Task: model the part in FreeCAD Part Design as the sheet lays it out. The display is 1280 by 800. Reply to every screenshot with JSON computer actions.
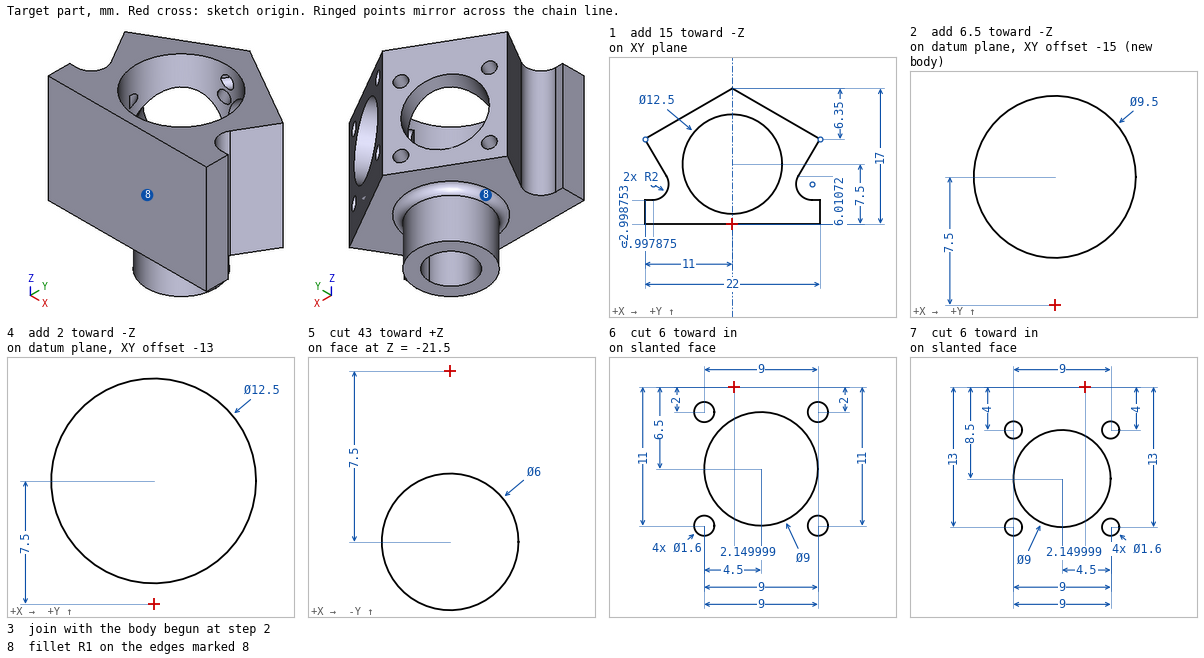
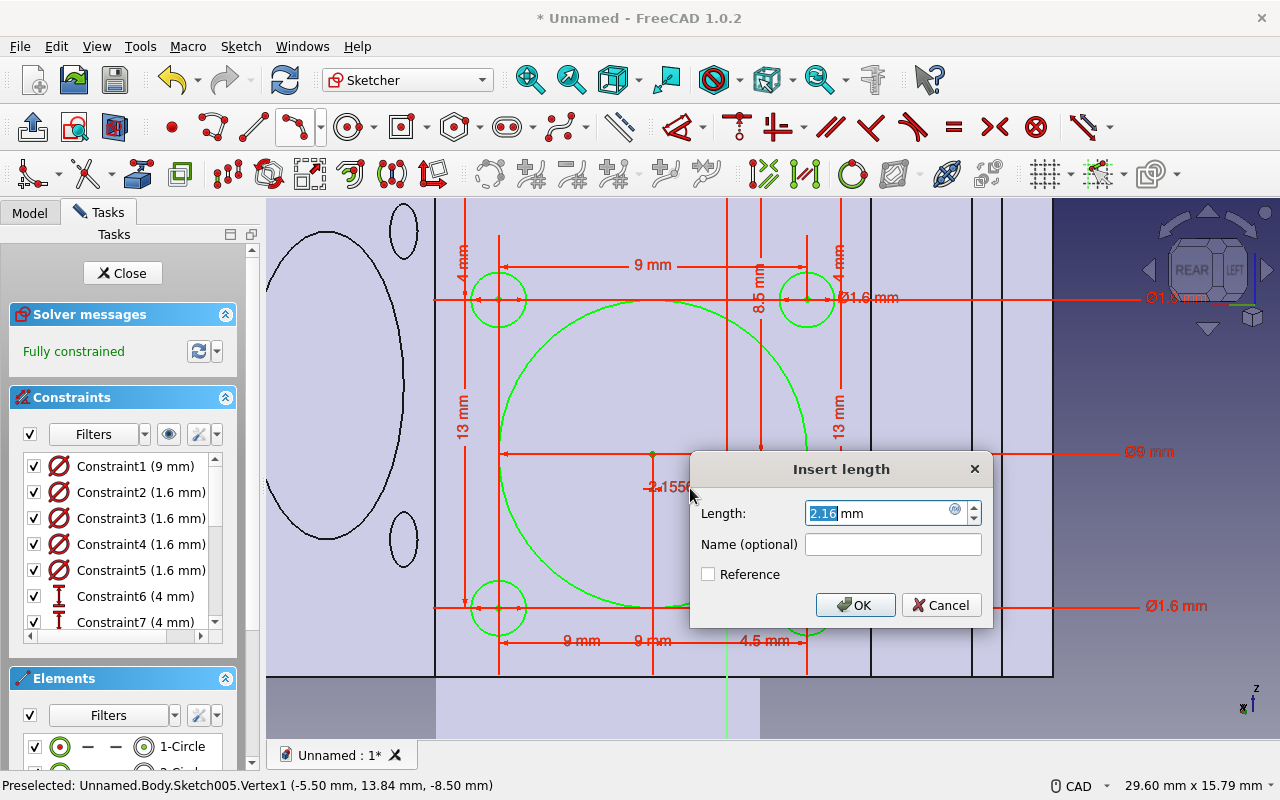
{"action": "type", "text": "2.149999"}
{"action": "key", "text": "Return"}
{"action": "key", "text": "Escape"}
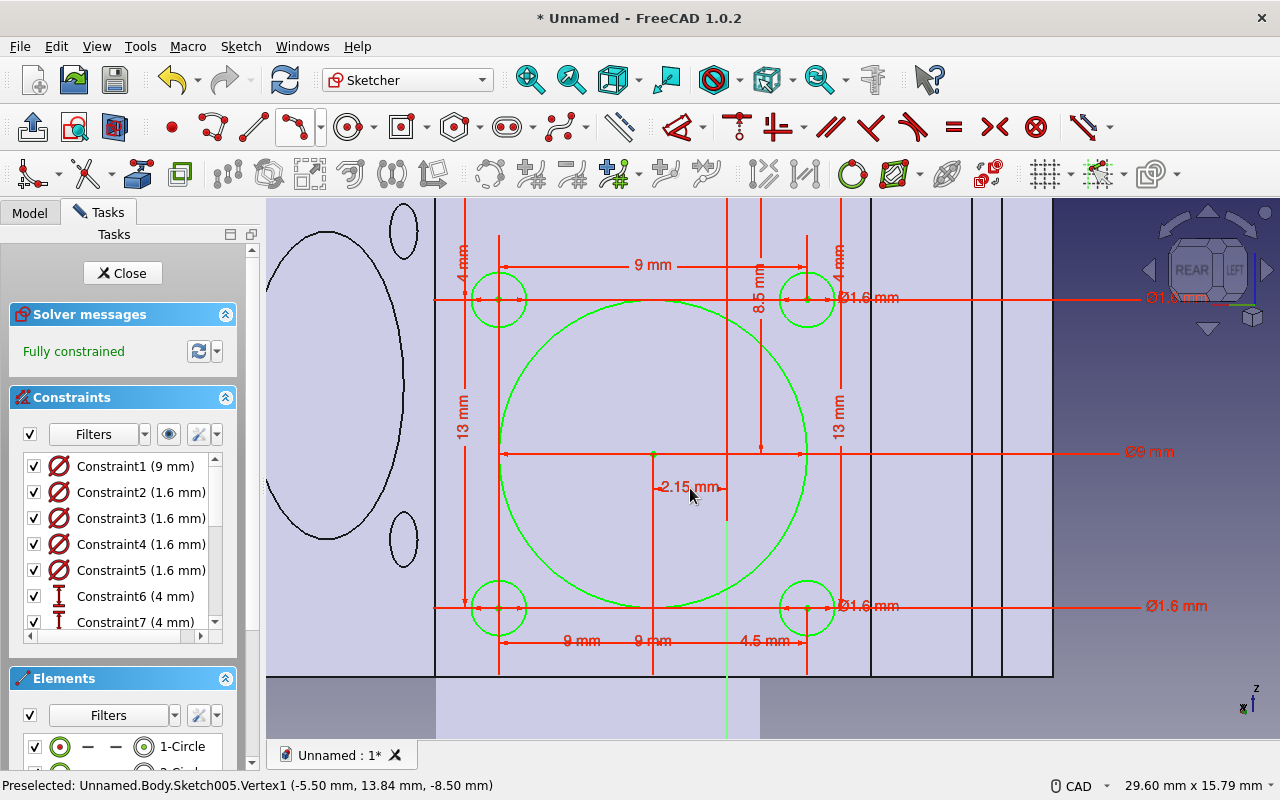
{"action": "left_click", "coordinate": [123, 273]}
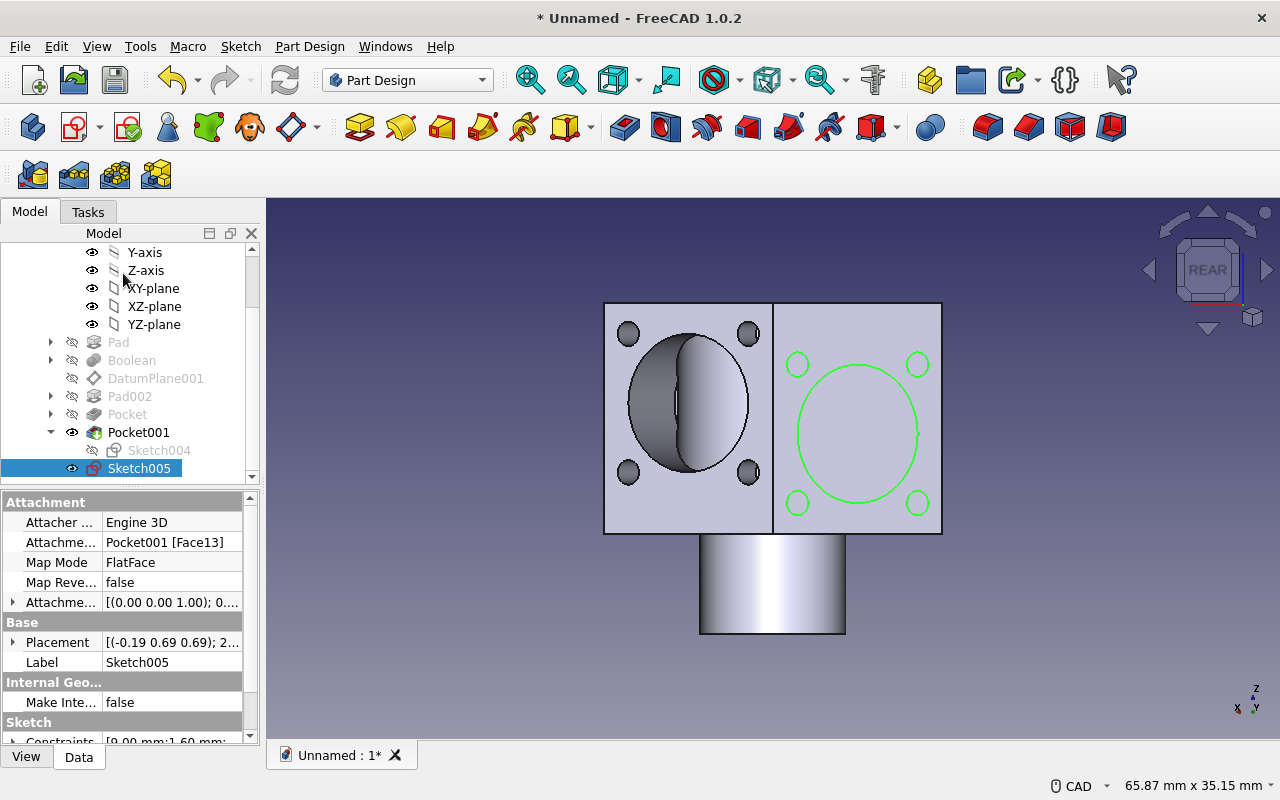
{"action": "left_click", "coordinate": [625, 128]}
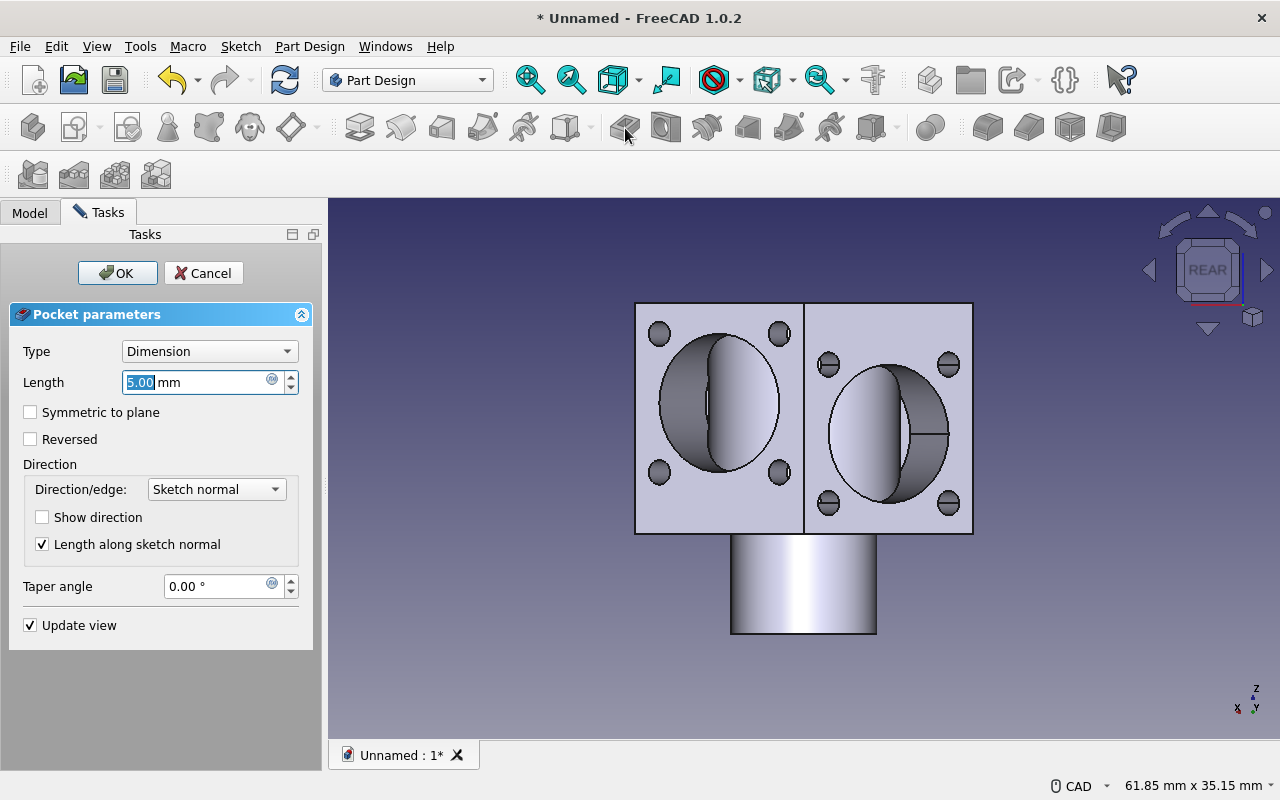
{"action": "type", "text": "6"}
{"action": "key", "text": "Tab"}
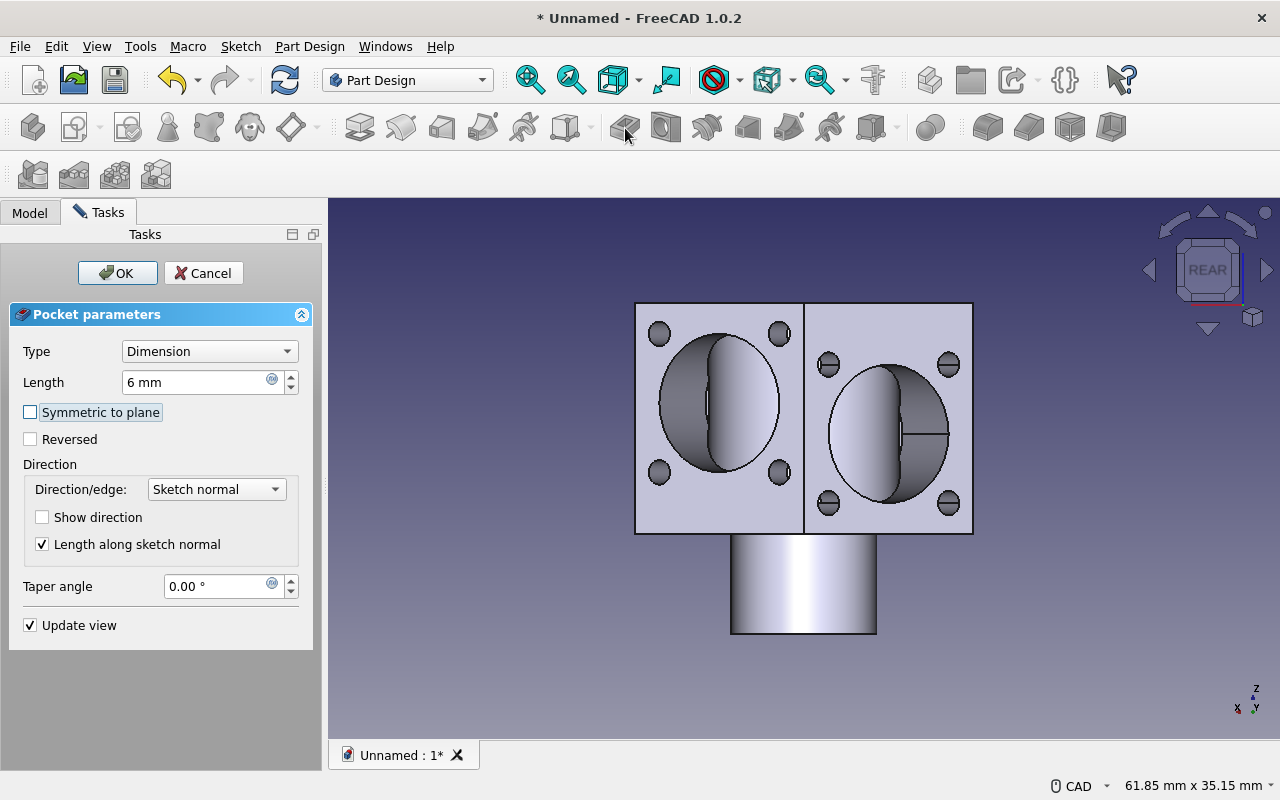
{"action": "left_click", "coordinate": [118, 273]}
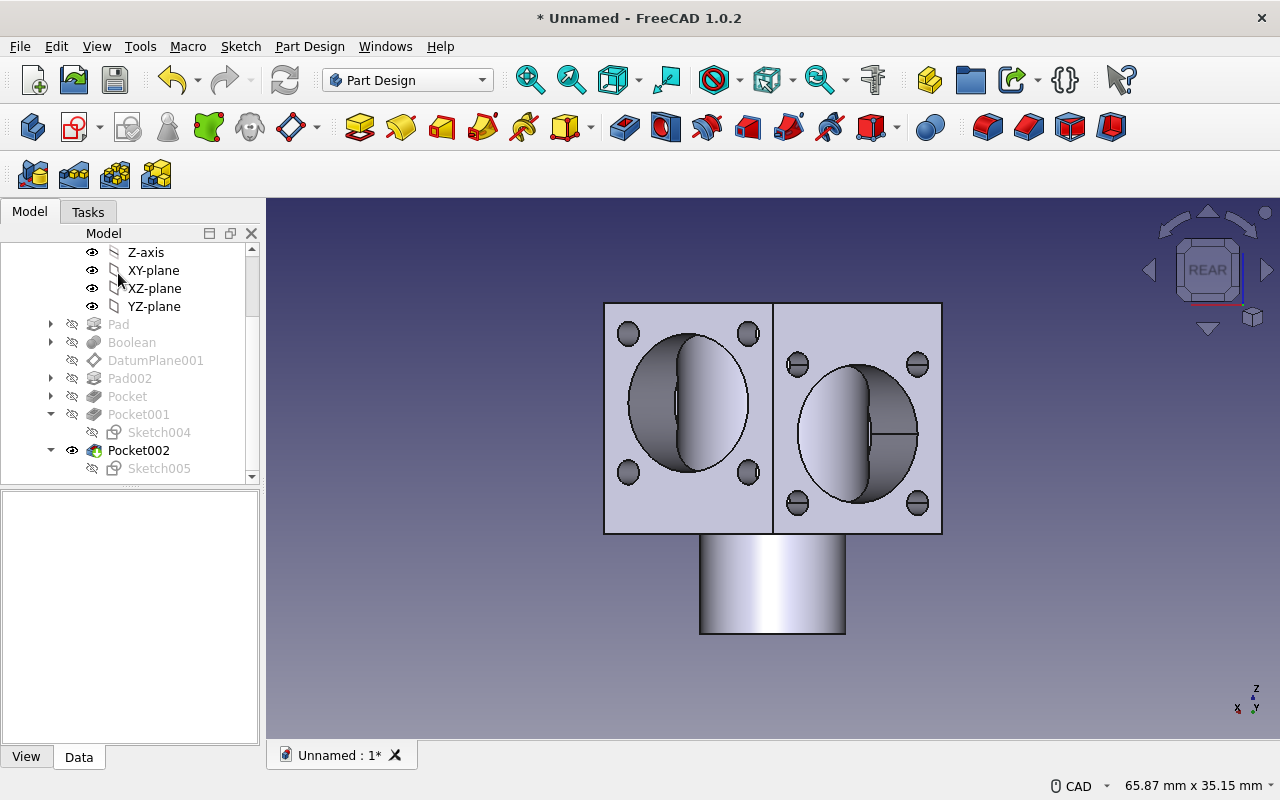
{"action": "key", "text": "0"}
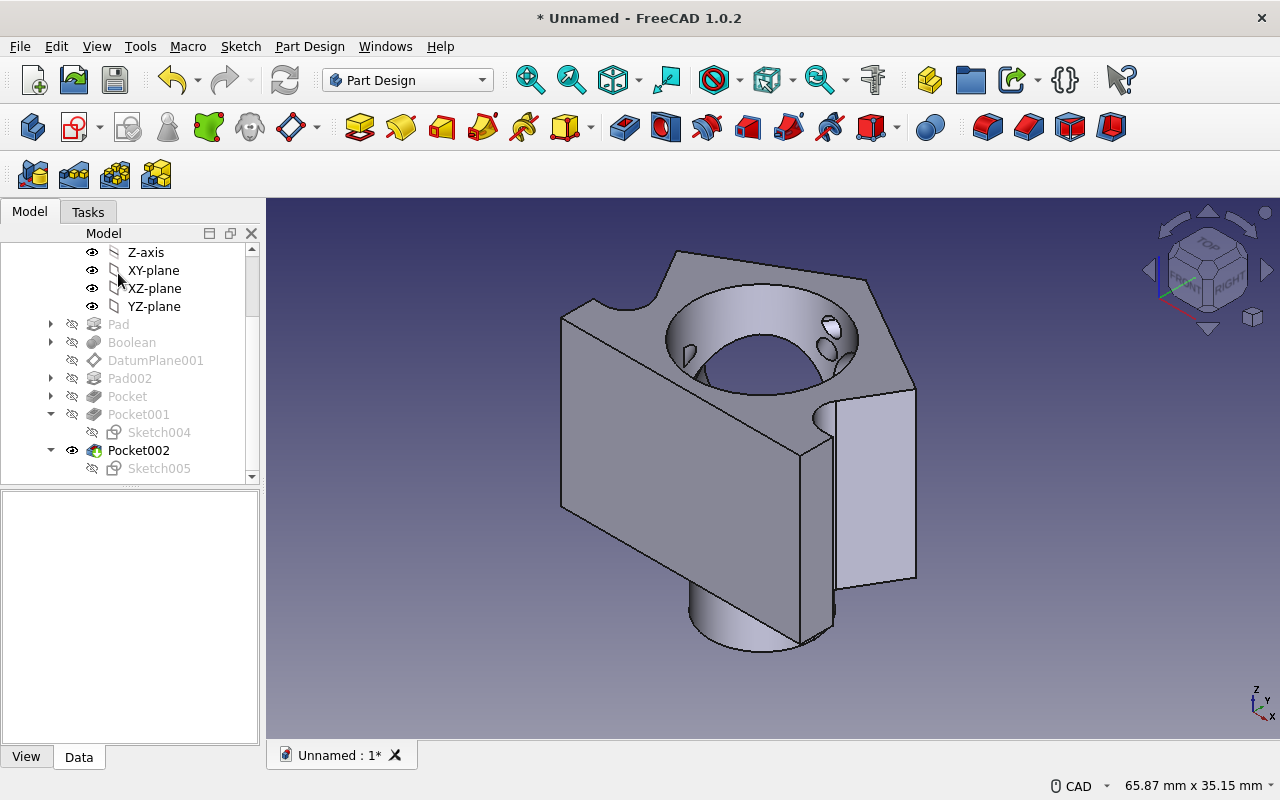
{"action": "key", "text": "2"}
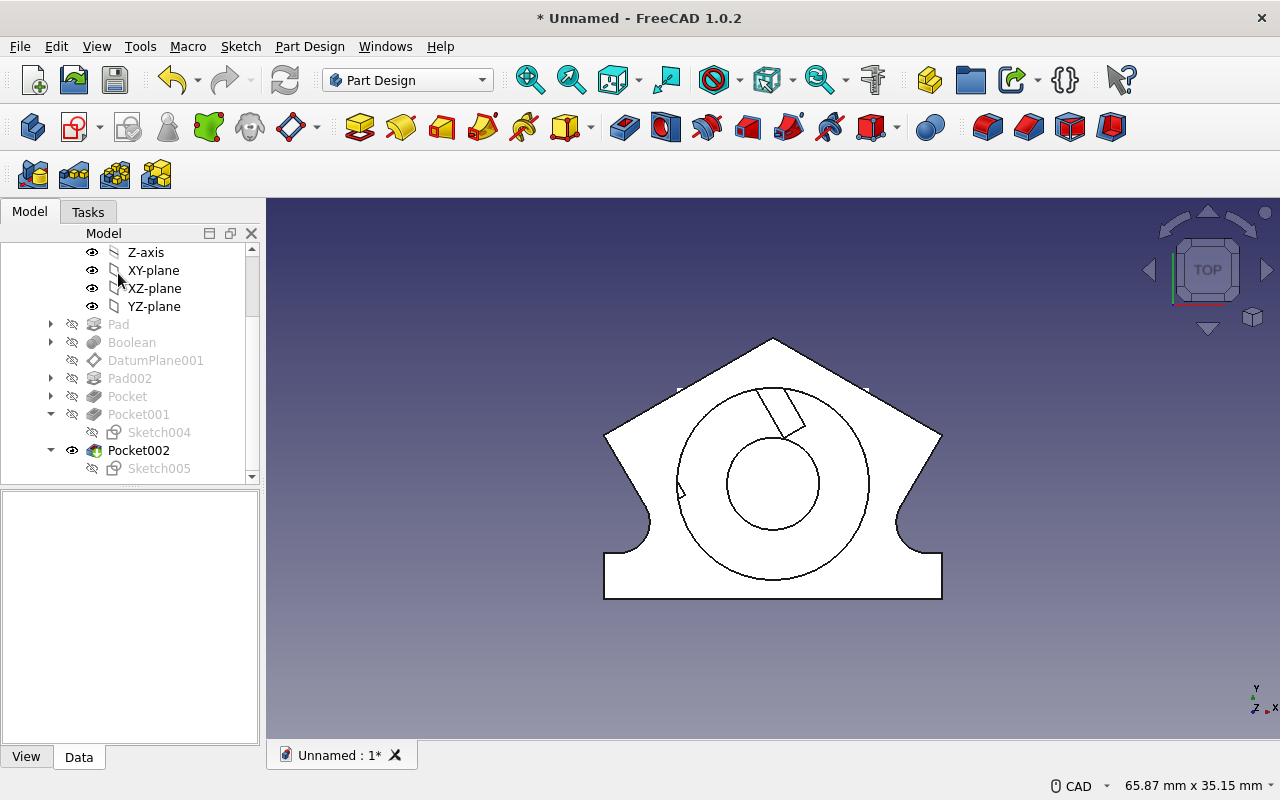
{"action": "key", "text": "1"}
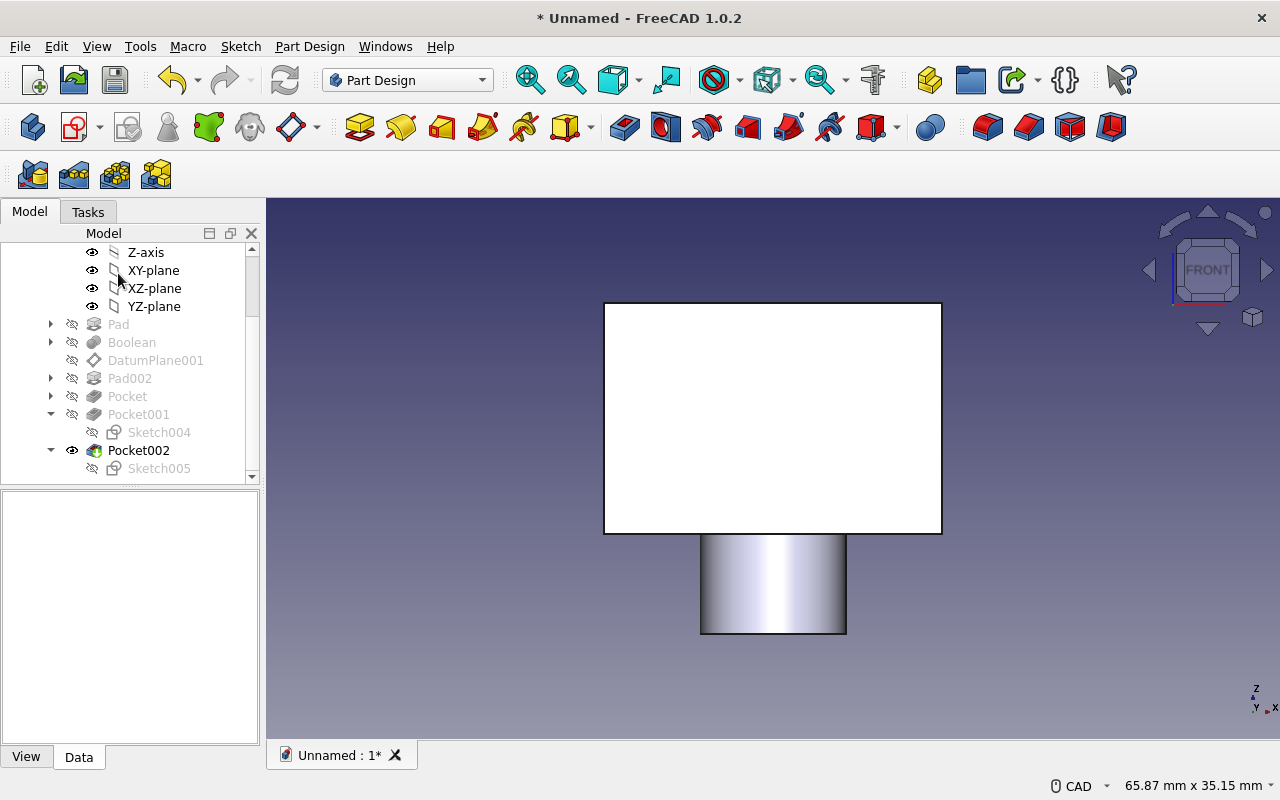
{"action": "key", "text": "3"}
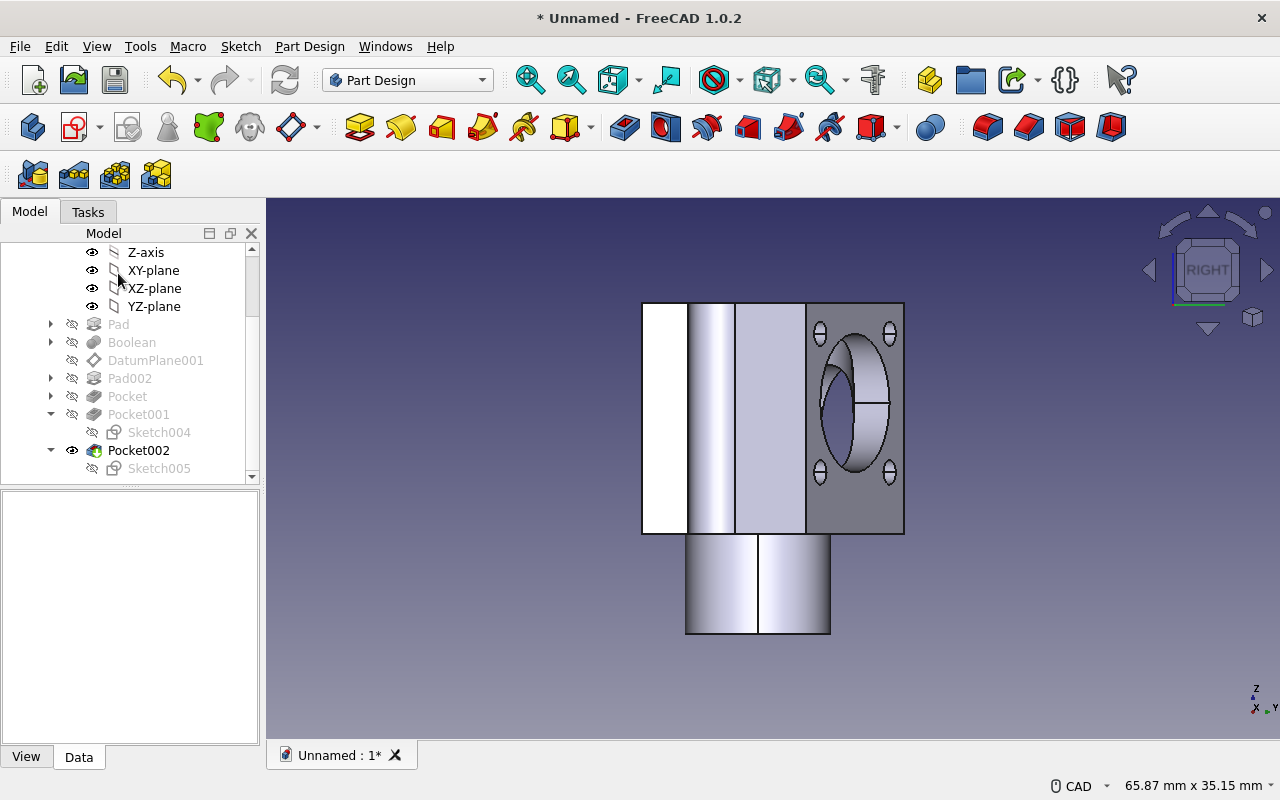
{"action": "key", "text": "5"}